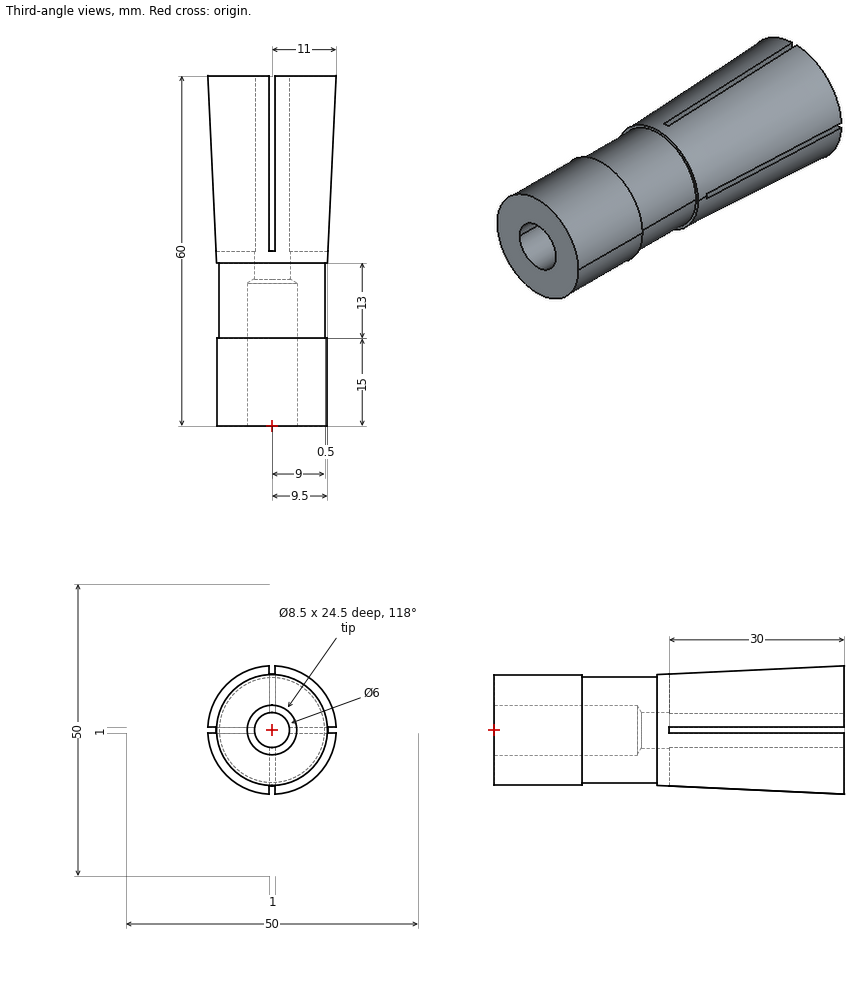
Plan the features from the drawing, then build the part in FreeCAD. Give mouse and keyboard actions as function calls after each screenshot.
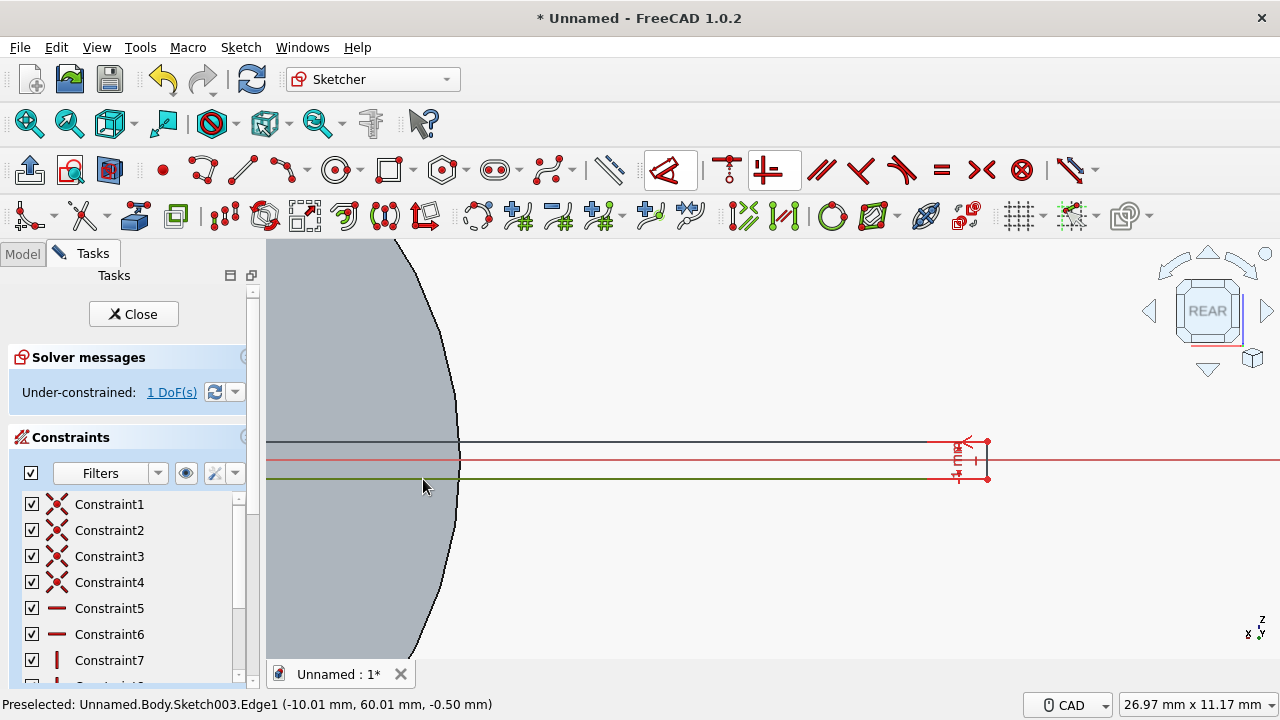
key(l)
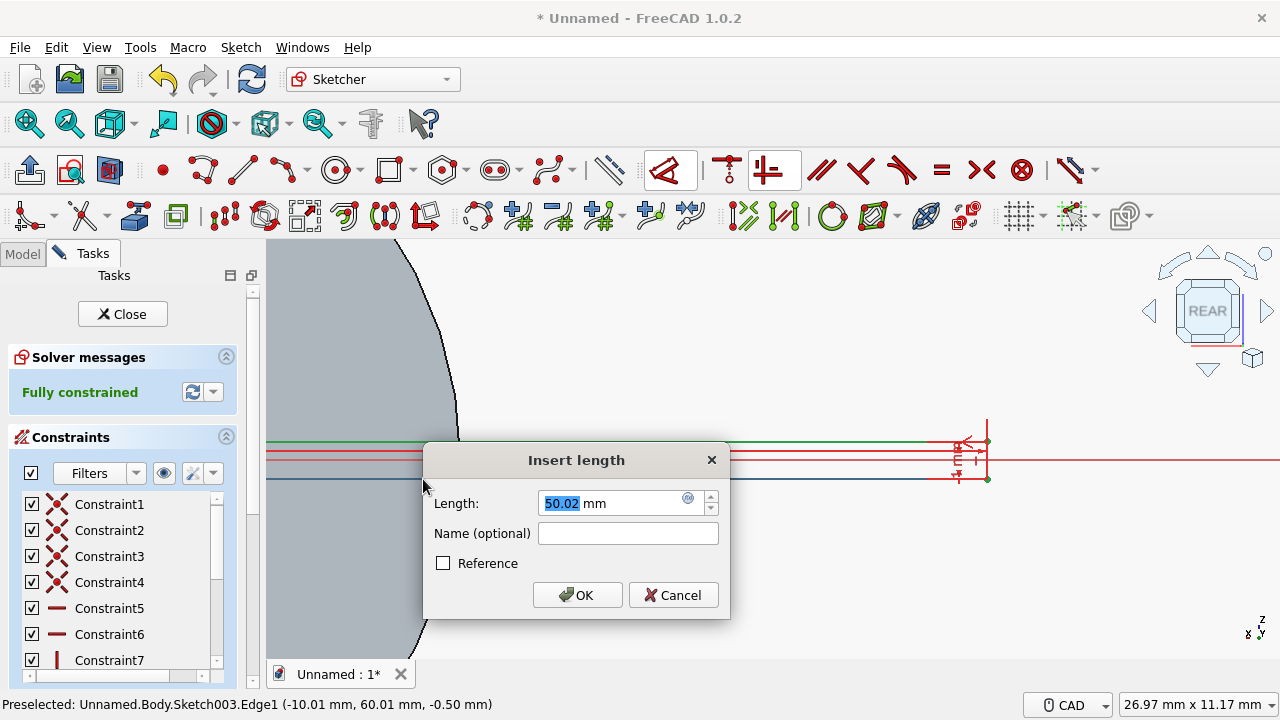
text(50)
key(Return)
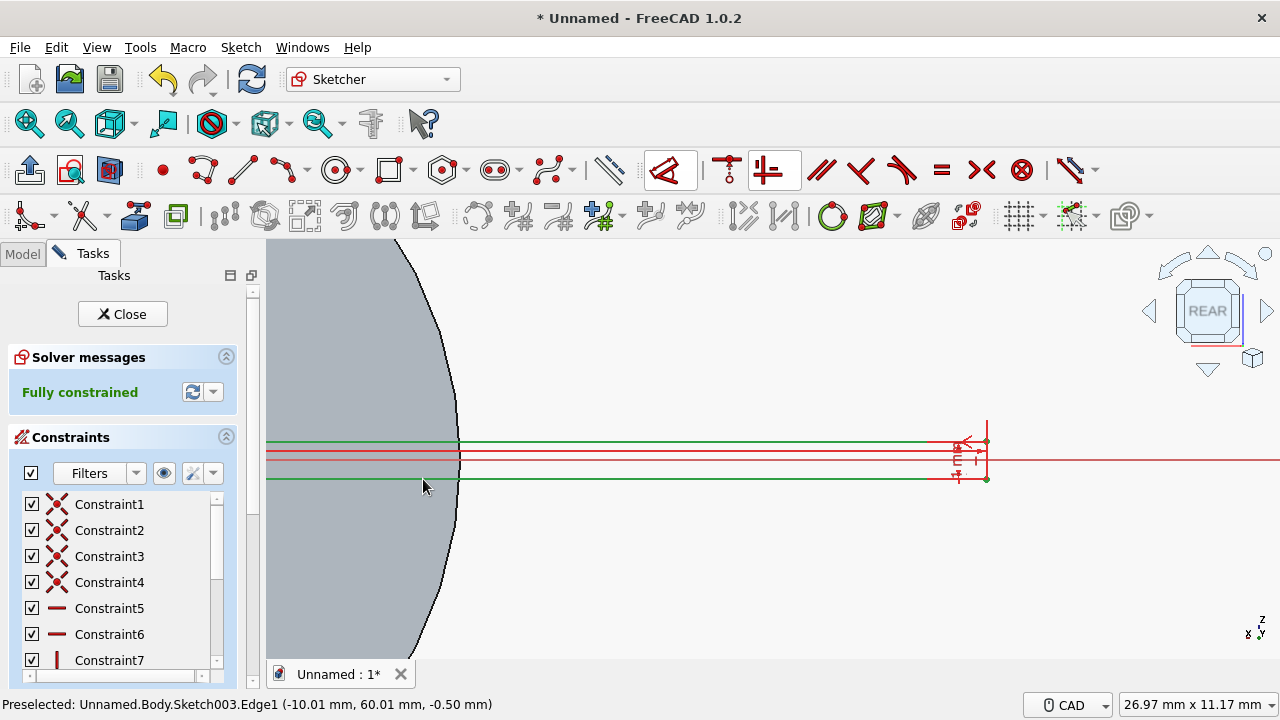
click(123, 314)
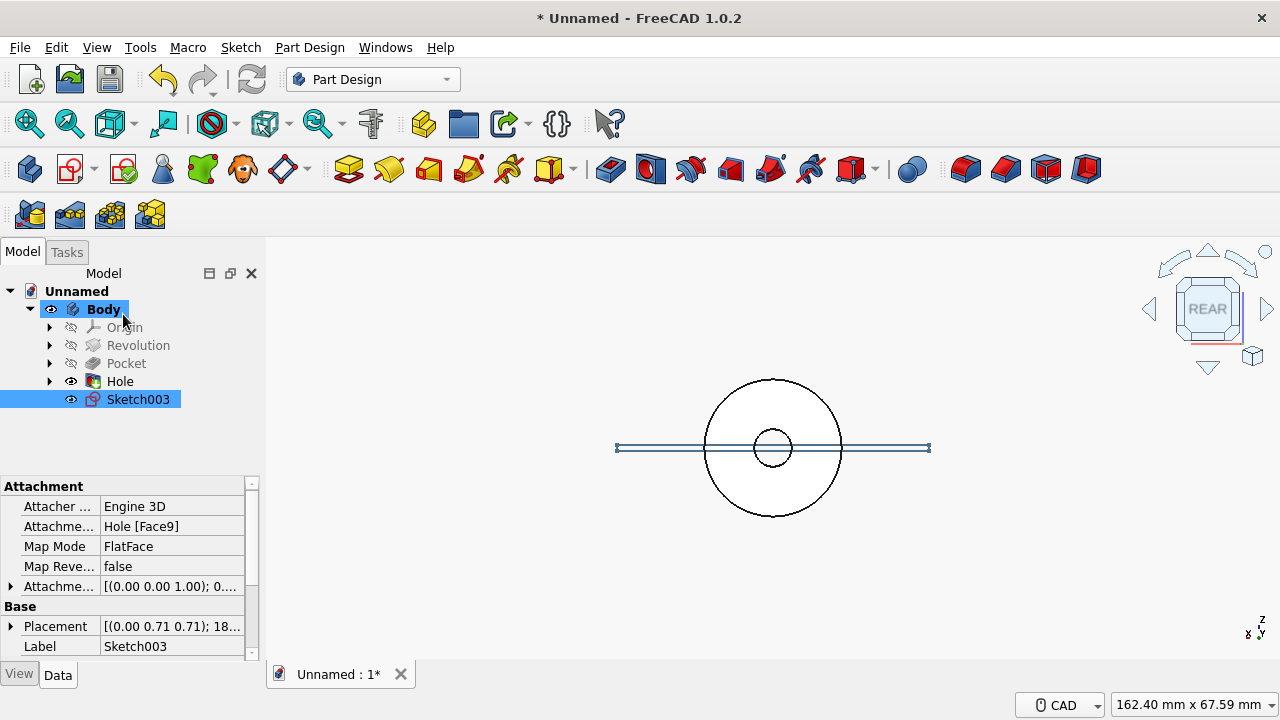
click(612, 170)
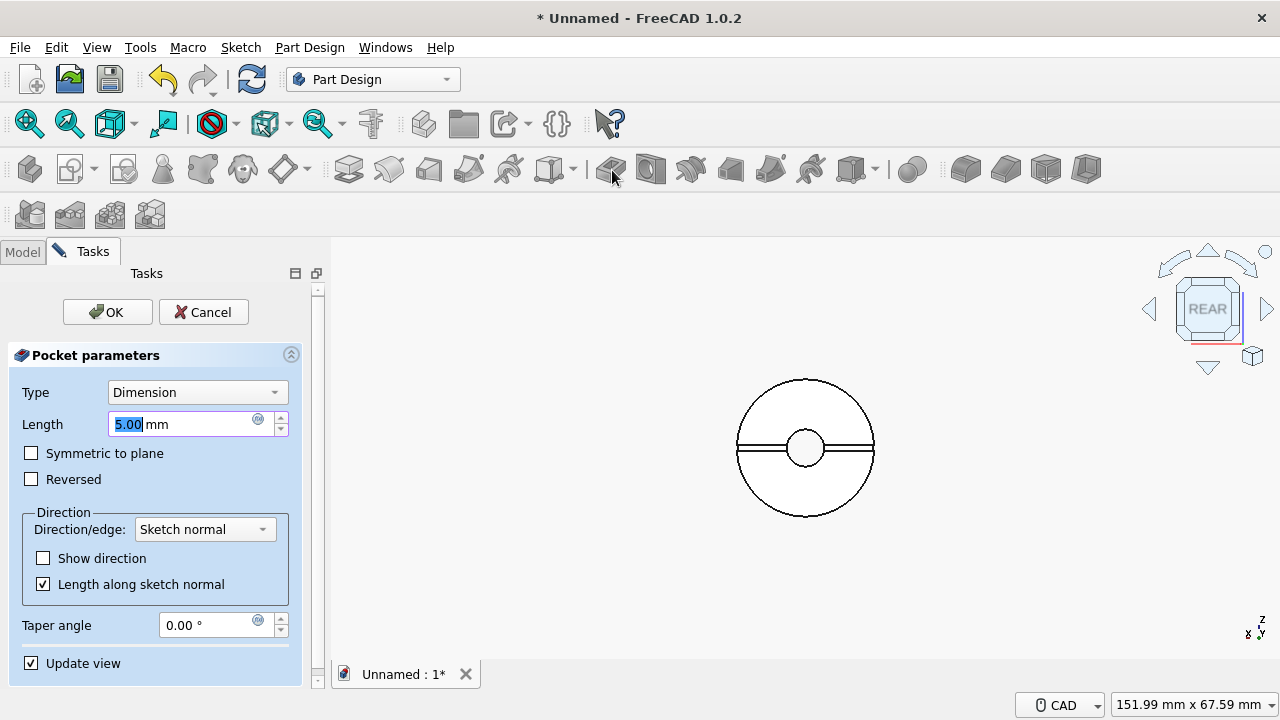
text(30)
key(Tab)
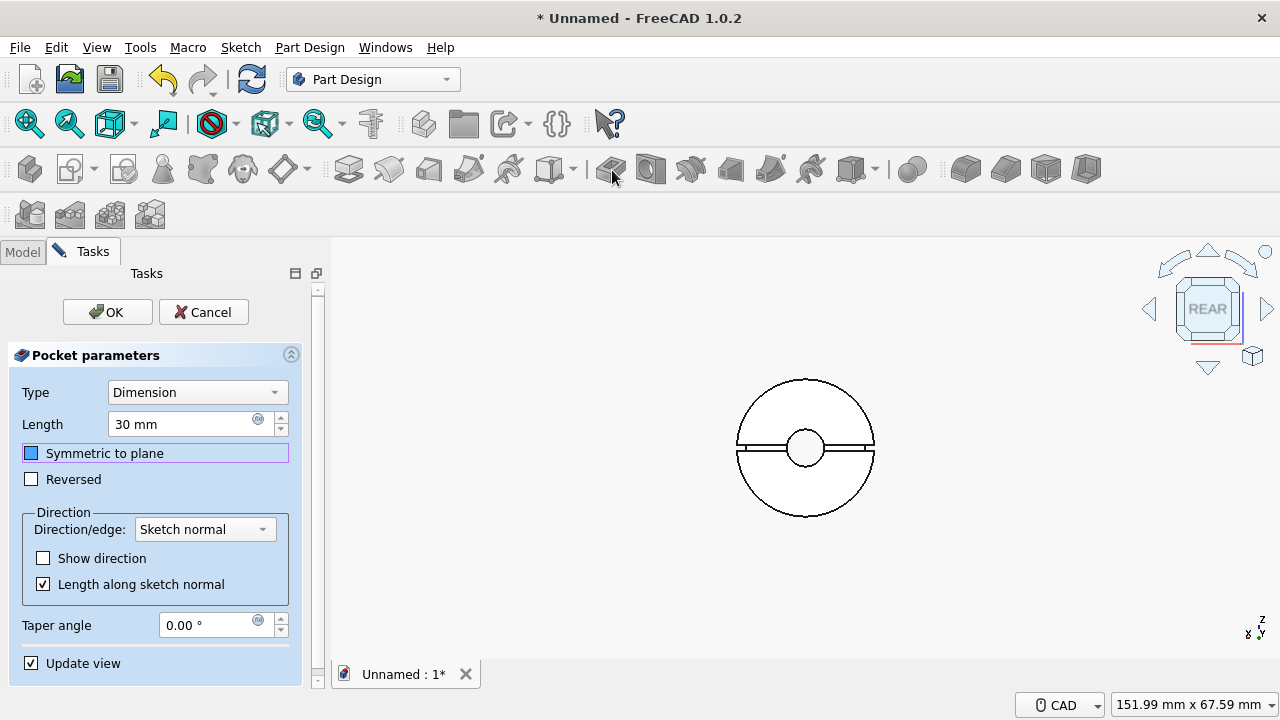
click(108, 312)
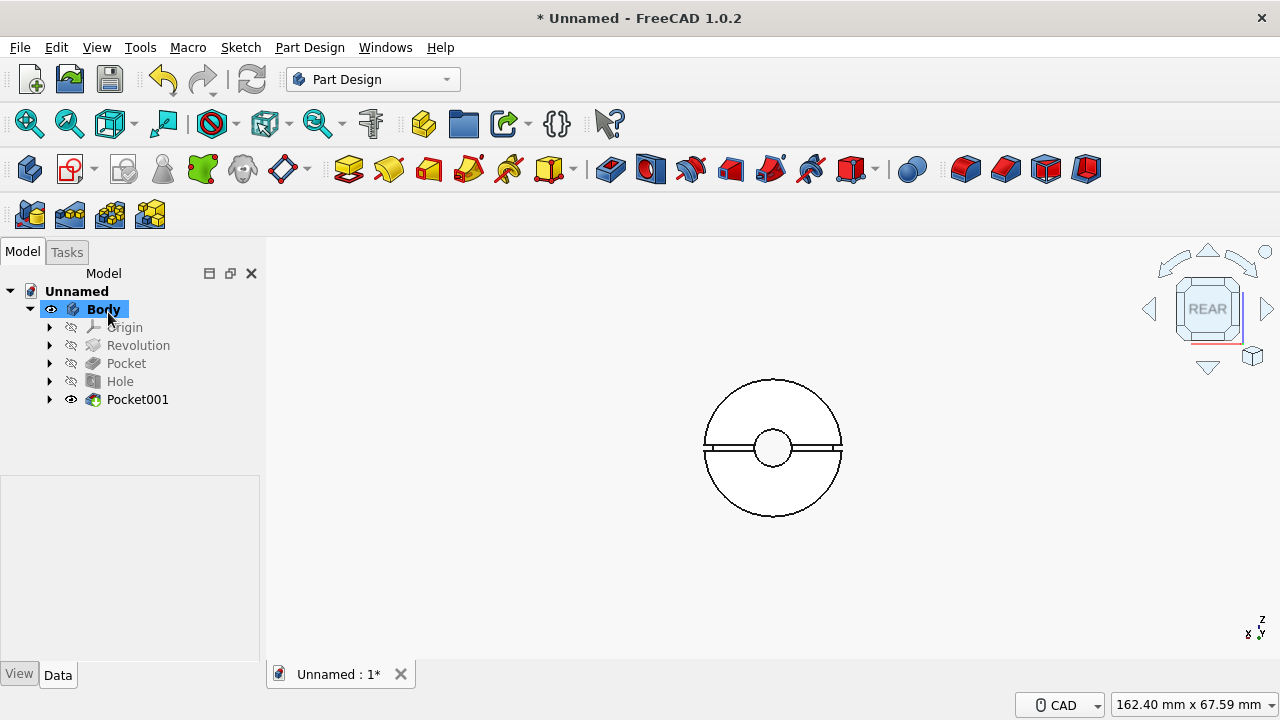
click(30, 124)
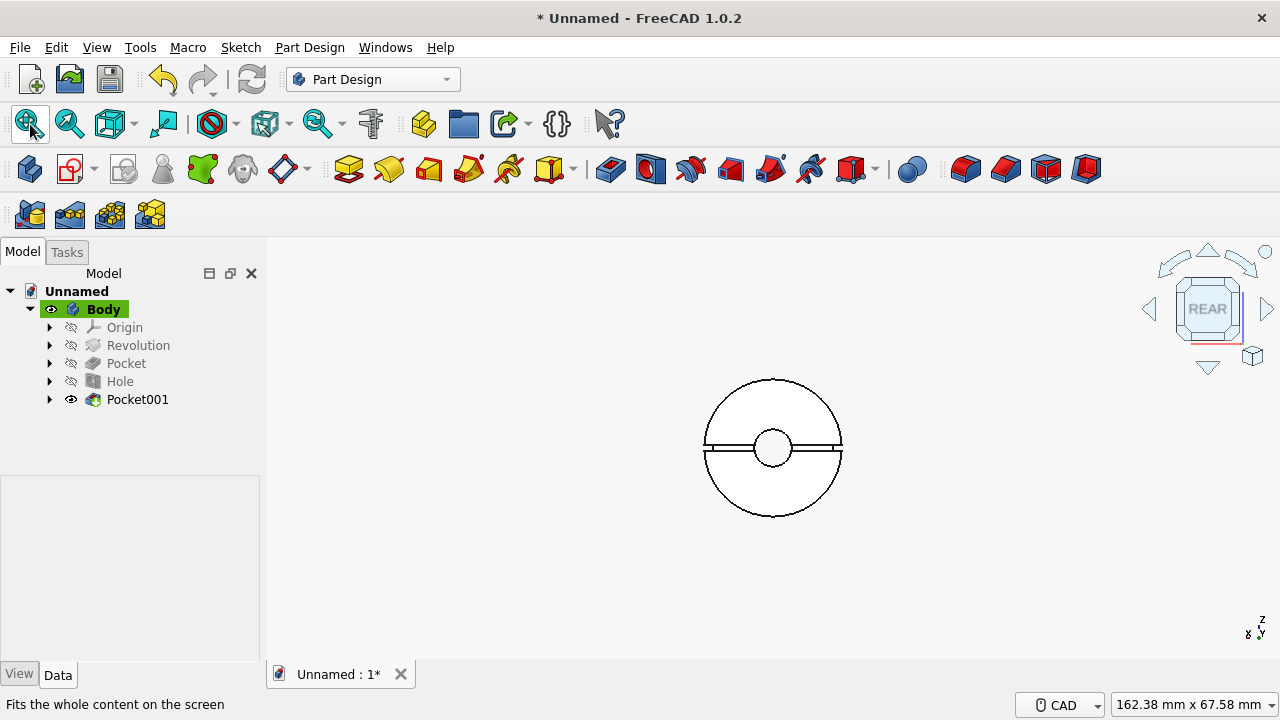
click(773, 402)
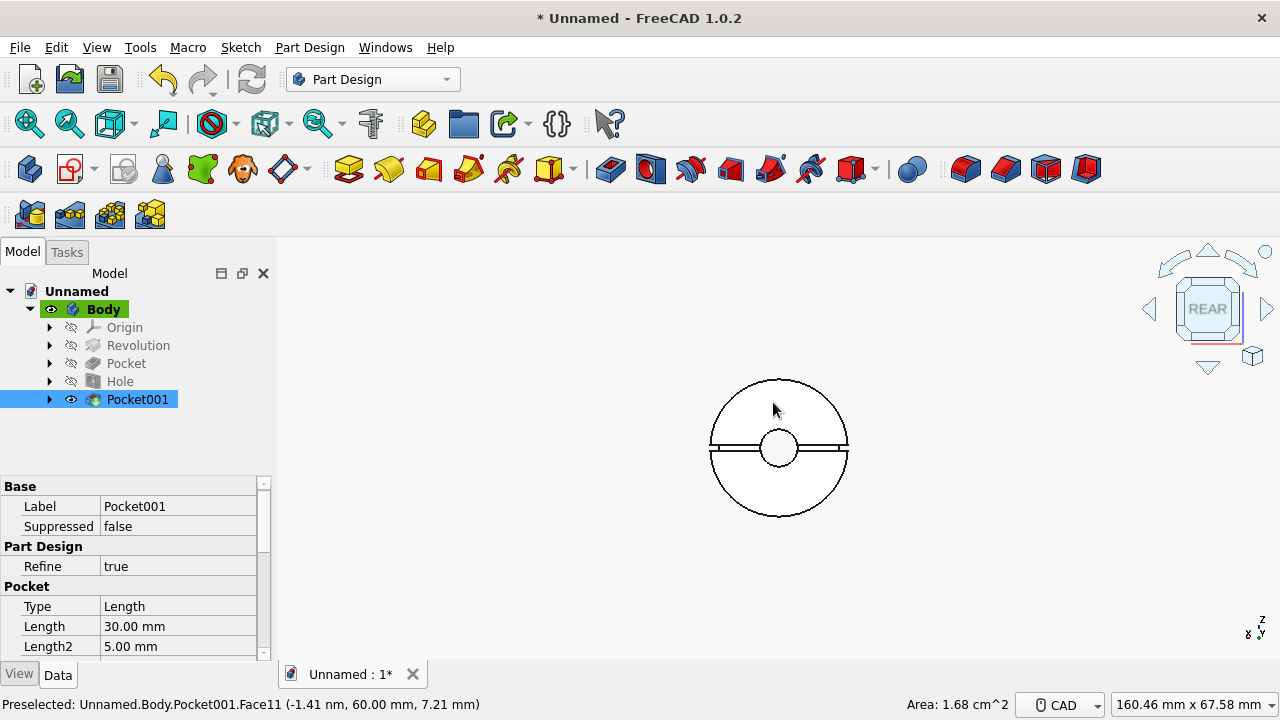
click(70, 170)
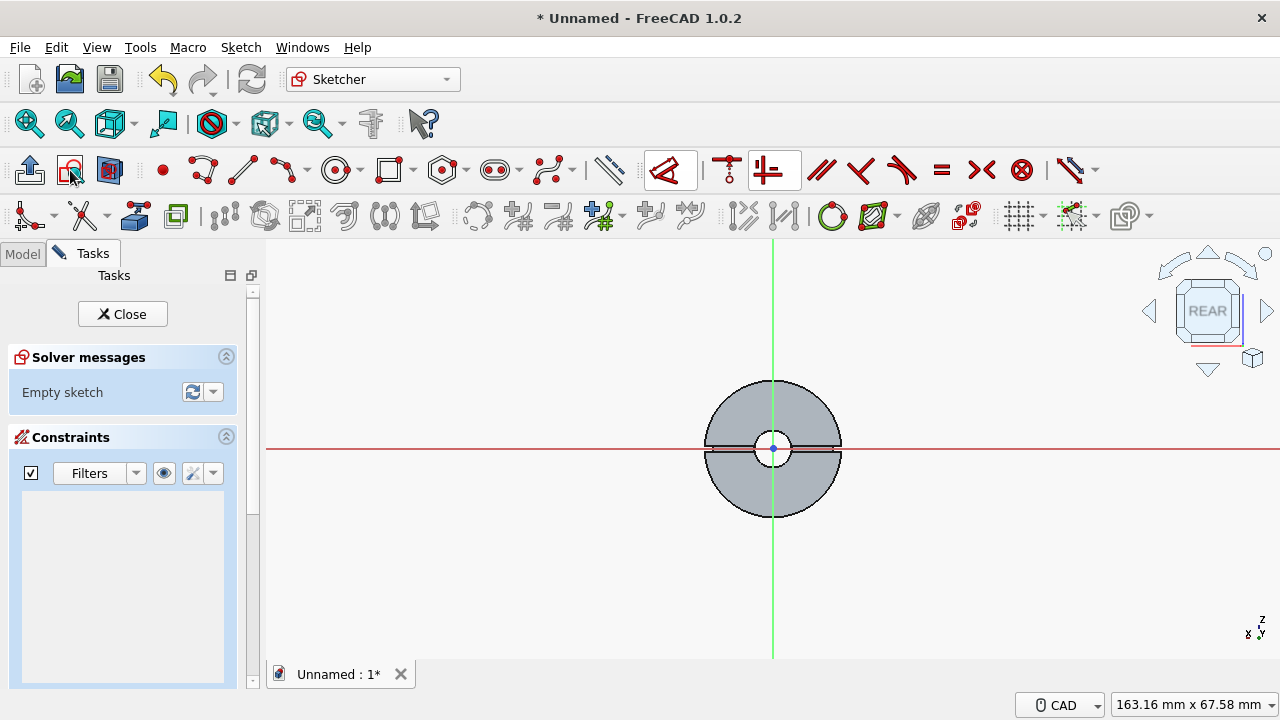
click(416, 170)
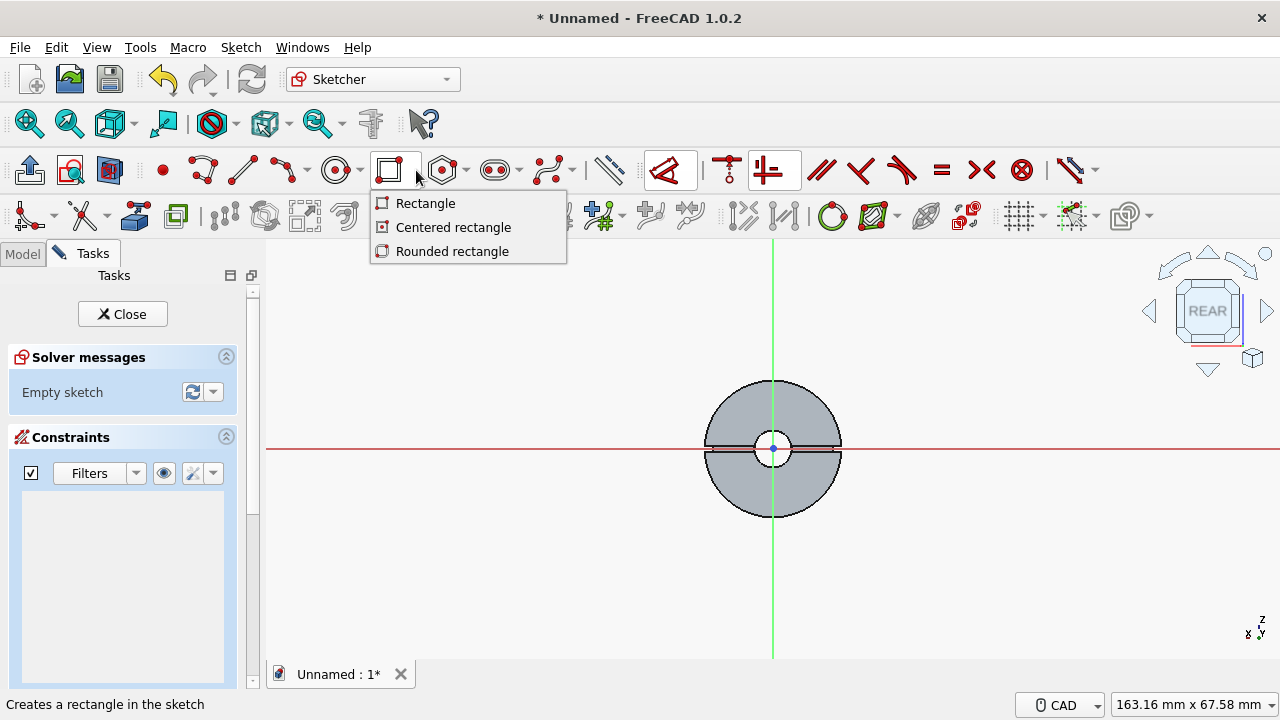
click(468, 227)